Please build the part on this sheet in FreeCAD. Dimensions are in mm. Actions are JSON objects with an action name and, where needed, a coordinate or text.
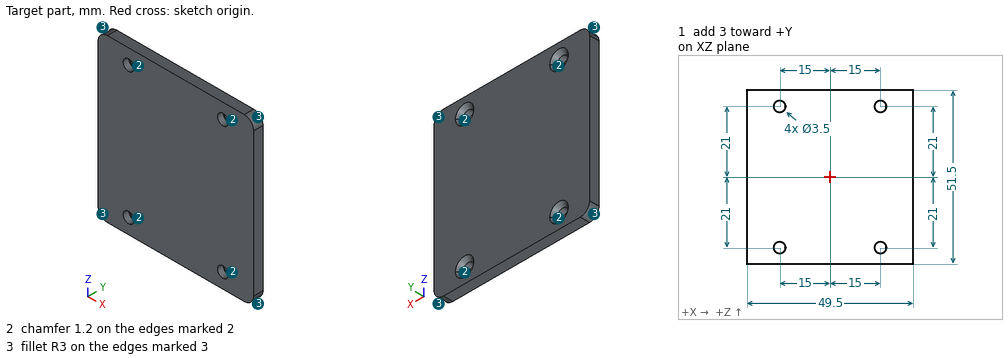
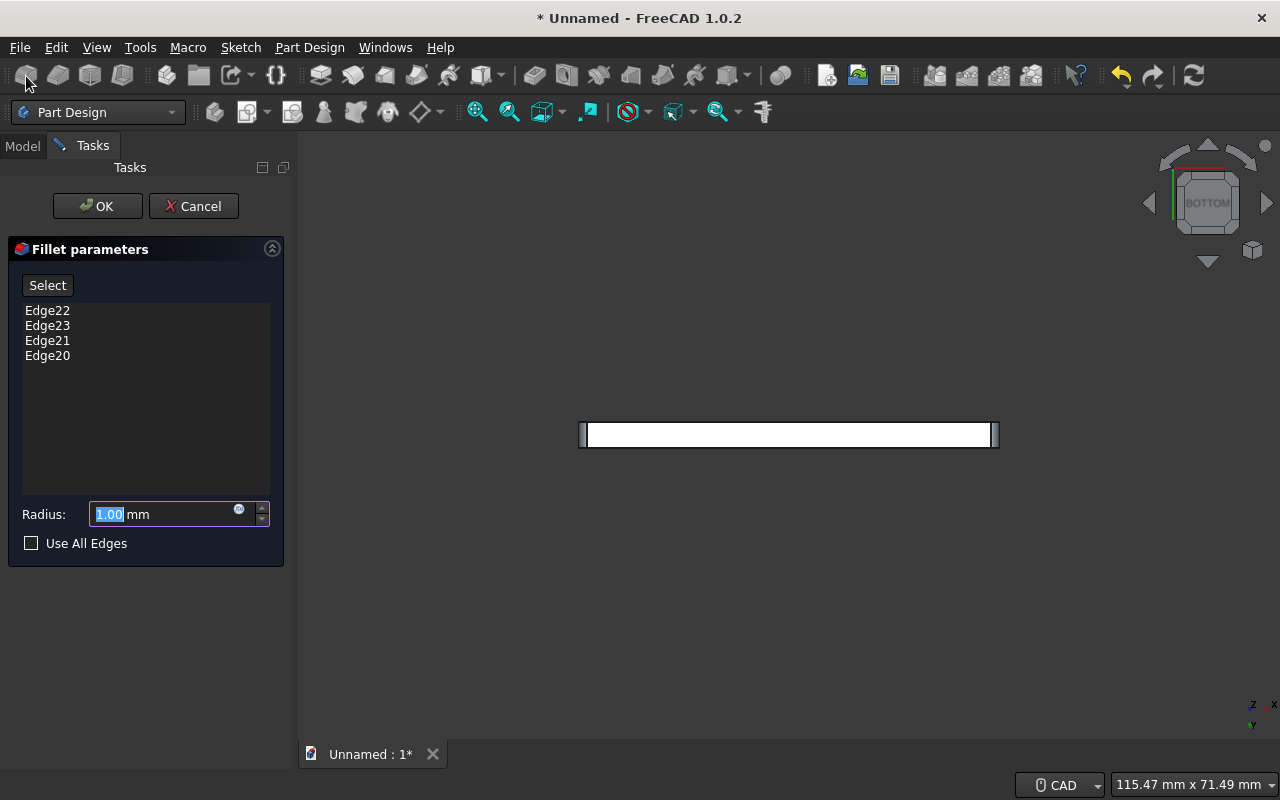
{"action": "type", "text": "3"}
{"action": "key", "text": "Tab"}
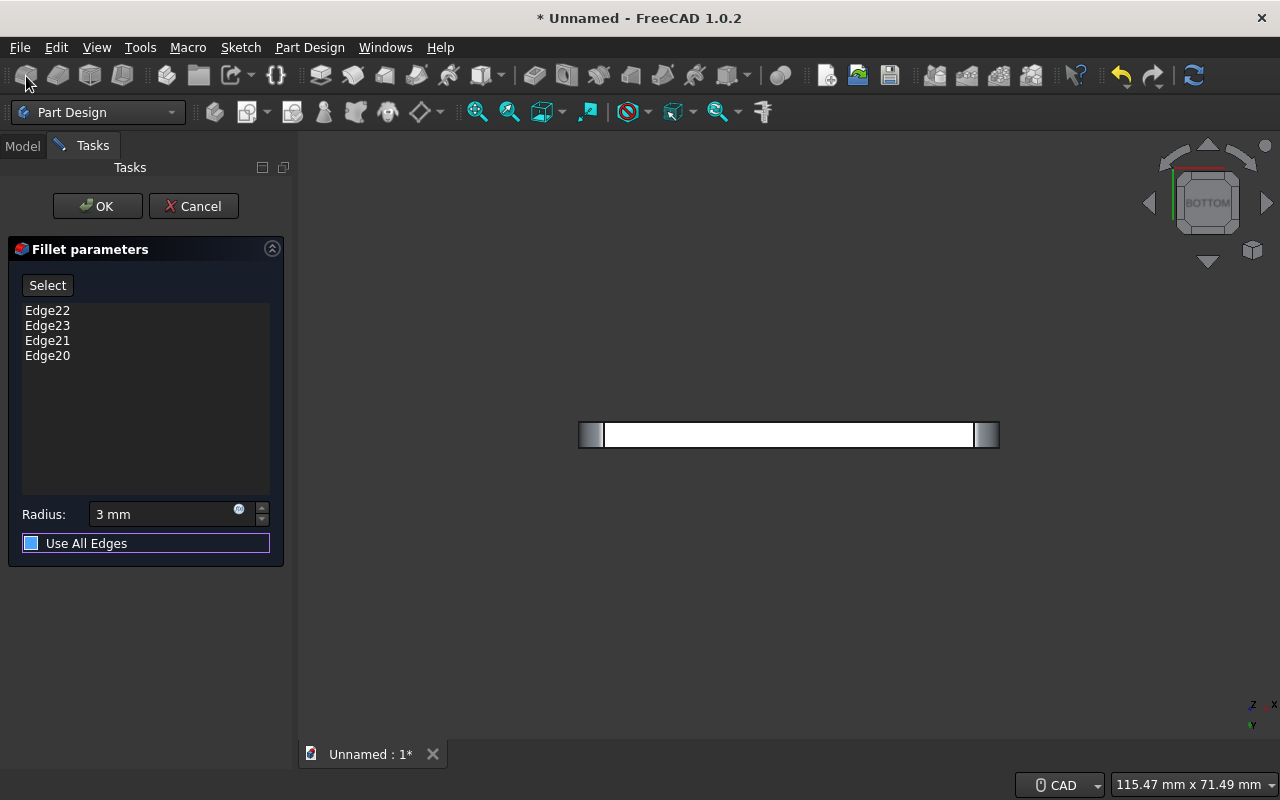
{"action": "left_click", "coordinate": [98, 206]}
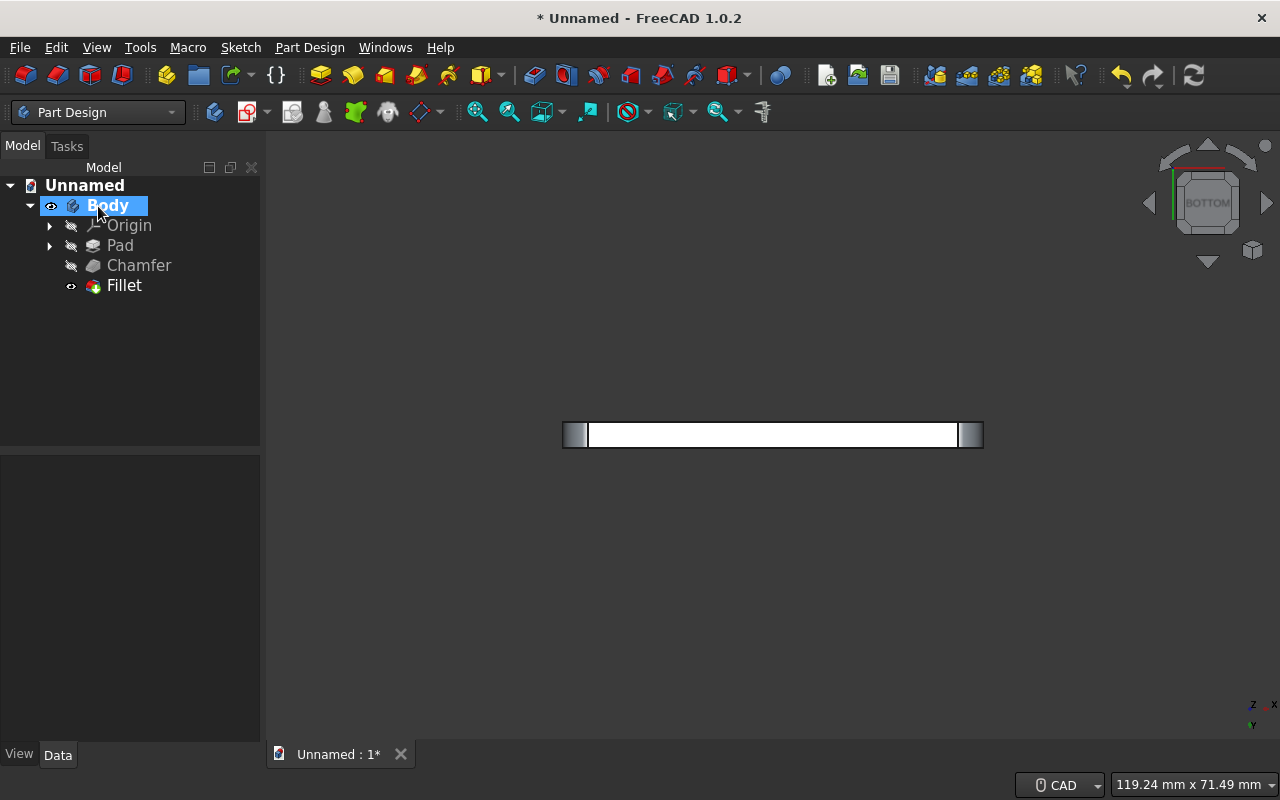
{"action": "key", "text": "0"}